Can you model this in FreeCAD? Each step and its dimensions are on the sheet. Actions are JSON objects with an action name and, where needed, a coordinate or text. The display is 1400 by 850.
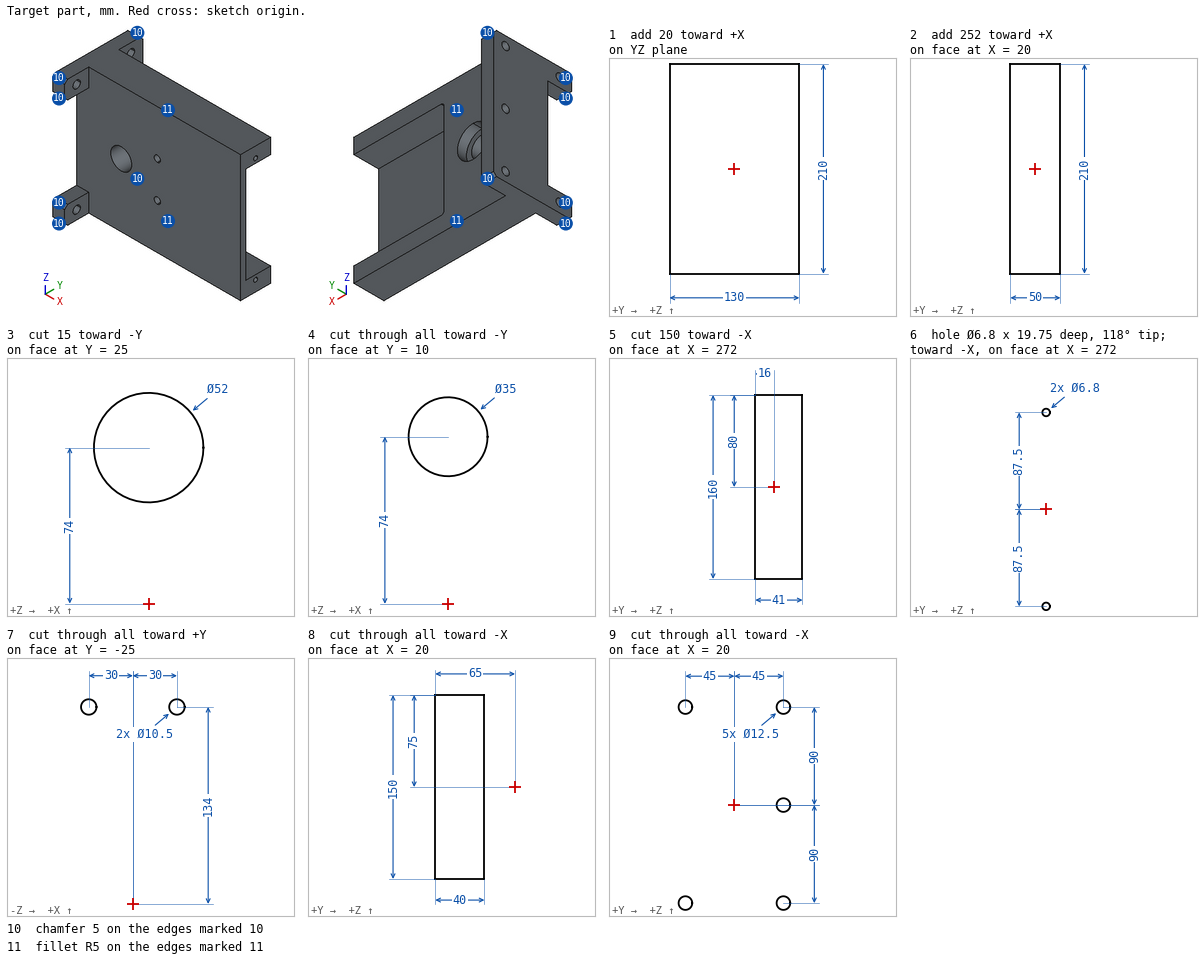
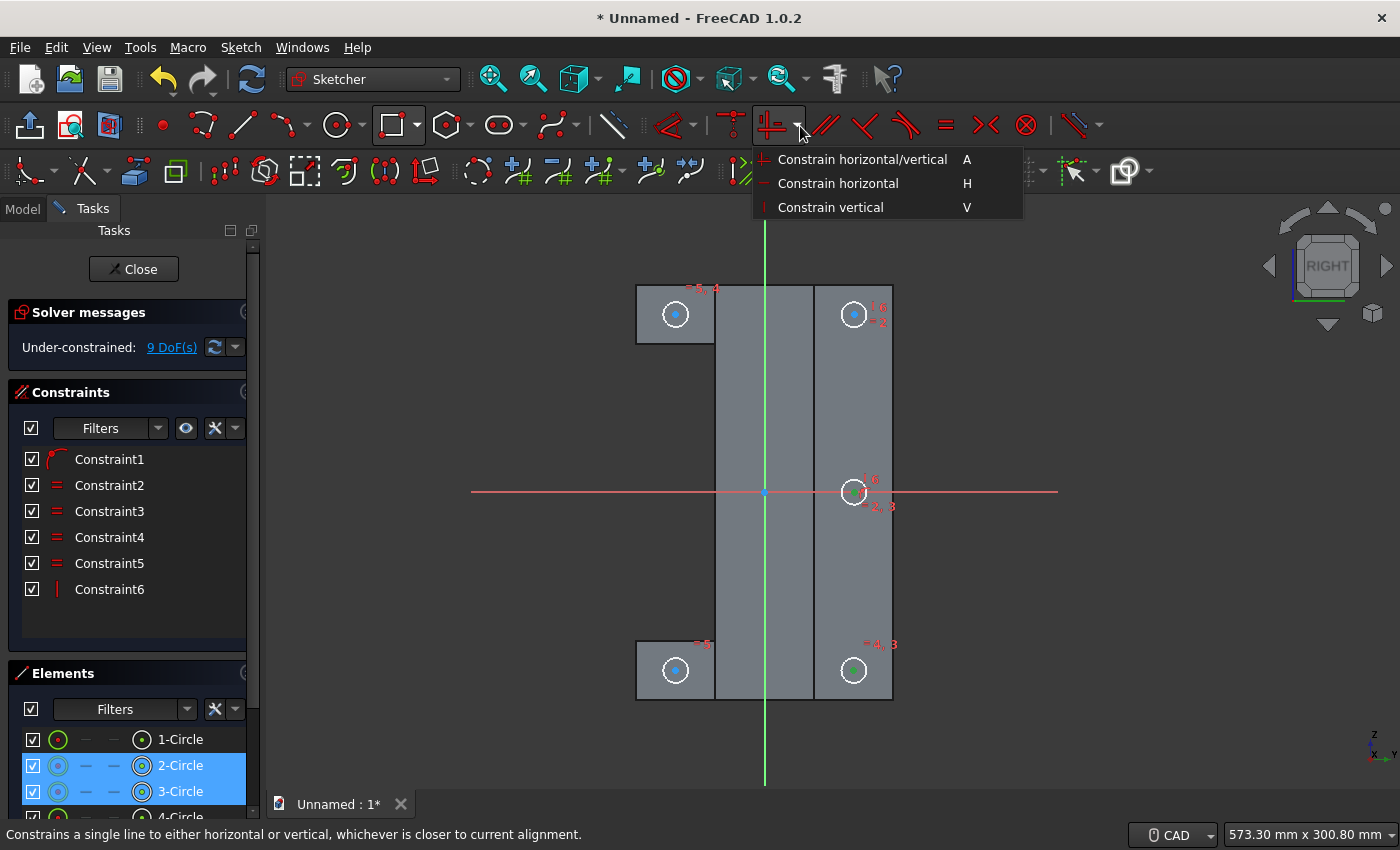
{"action": "left_click", "coordinate": [888, 207]}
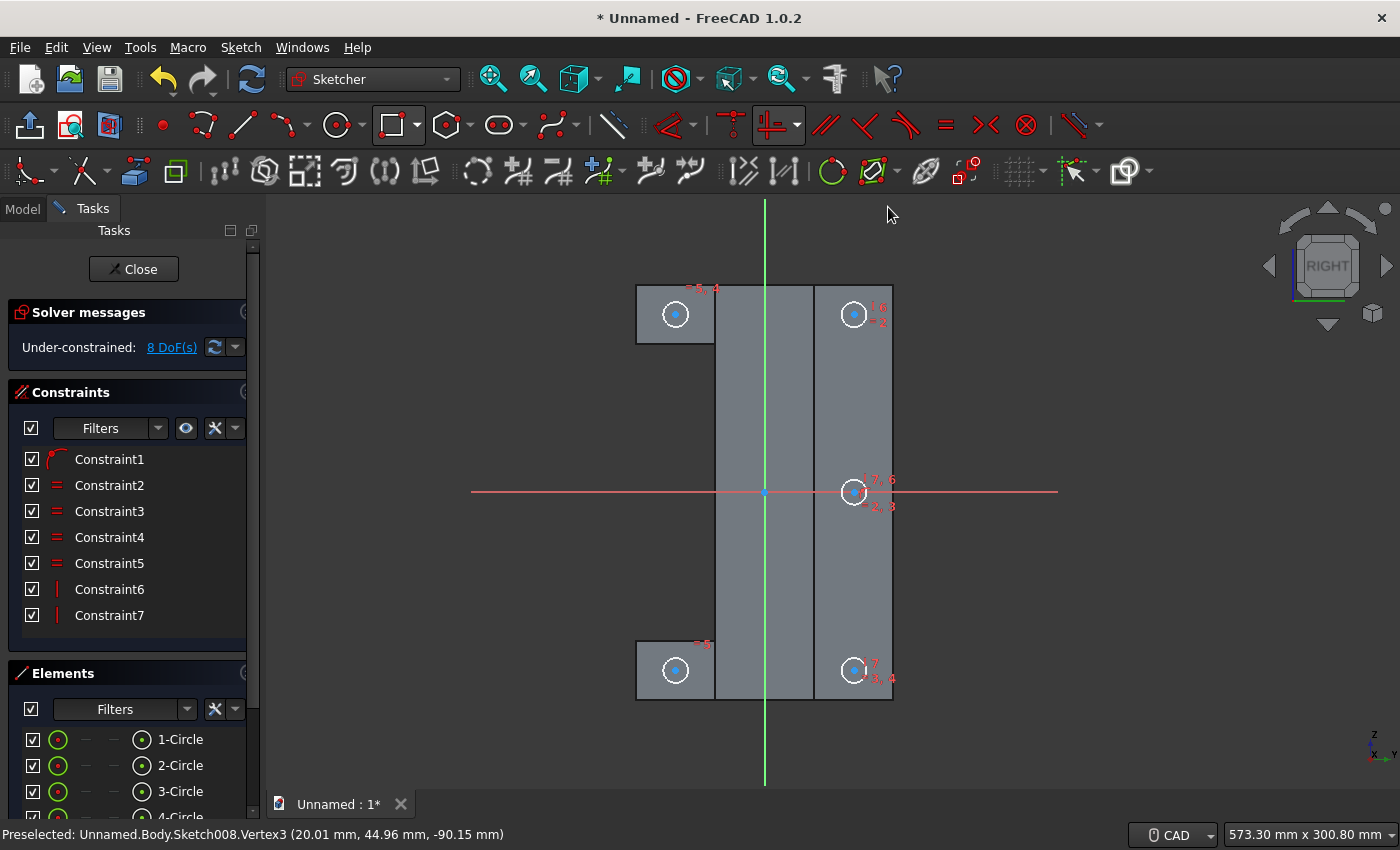
{"action": "left_click", "coordinate": [854, 315]}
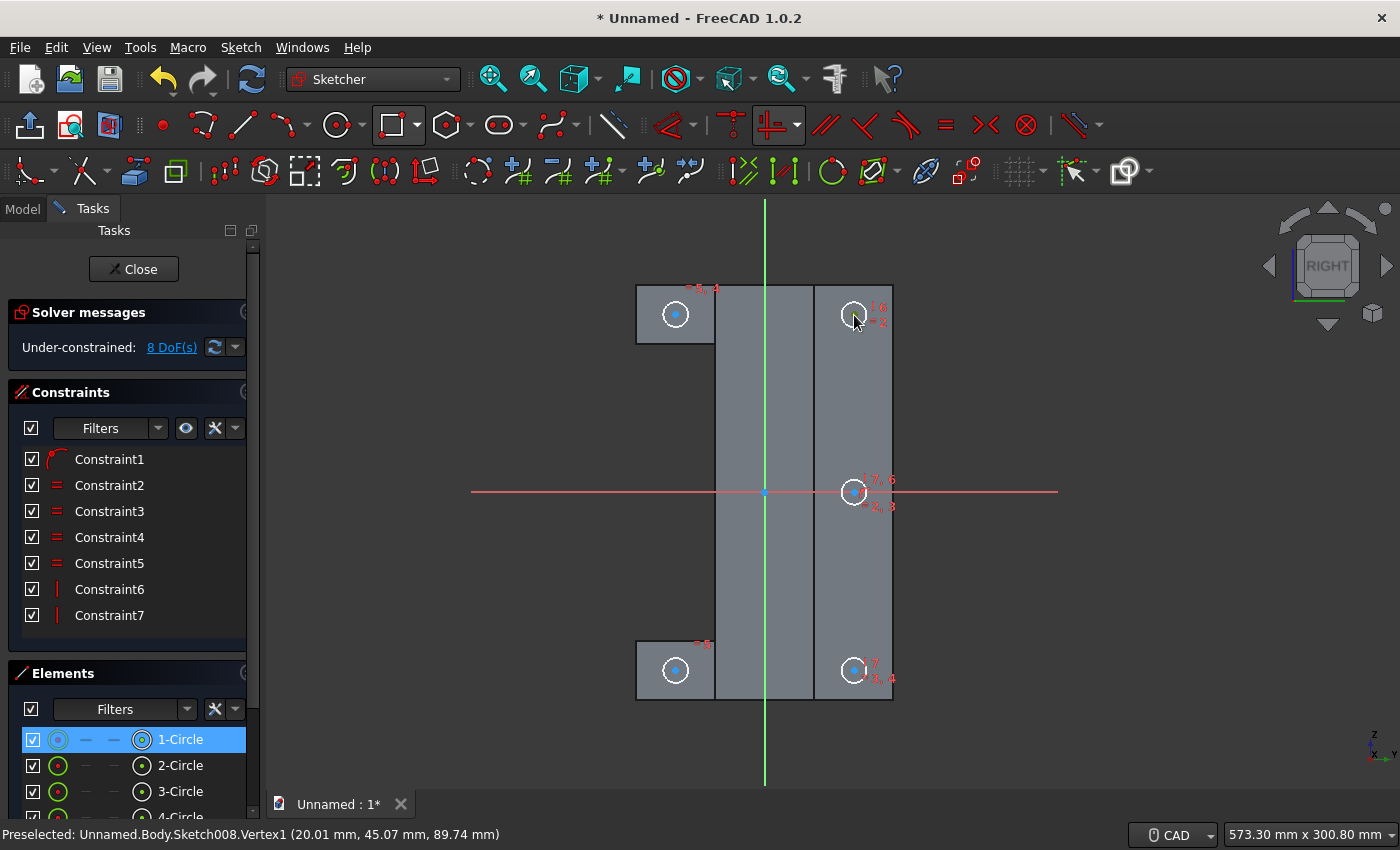
{"action": "left_click", "coordinate": [676, 315]}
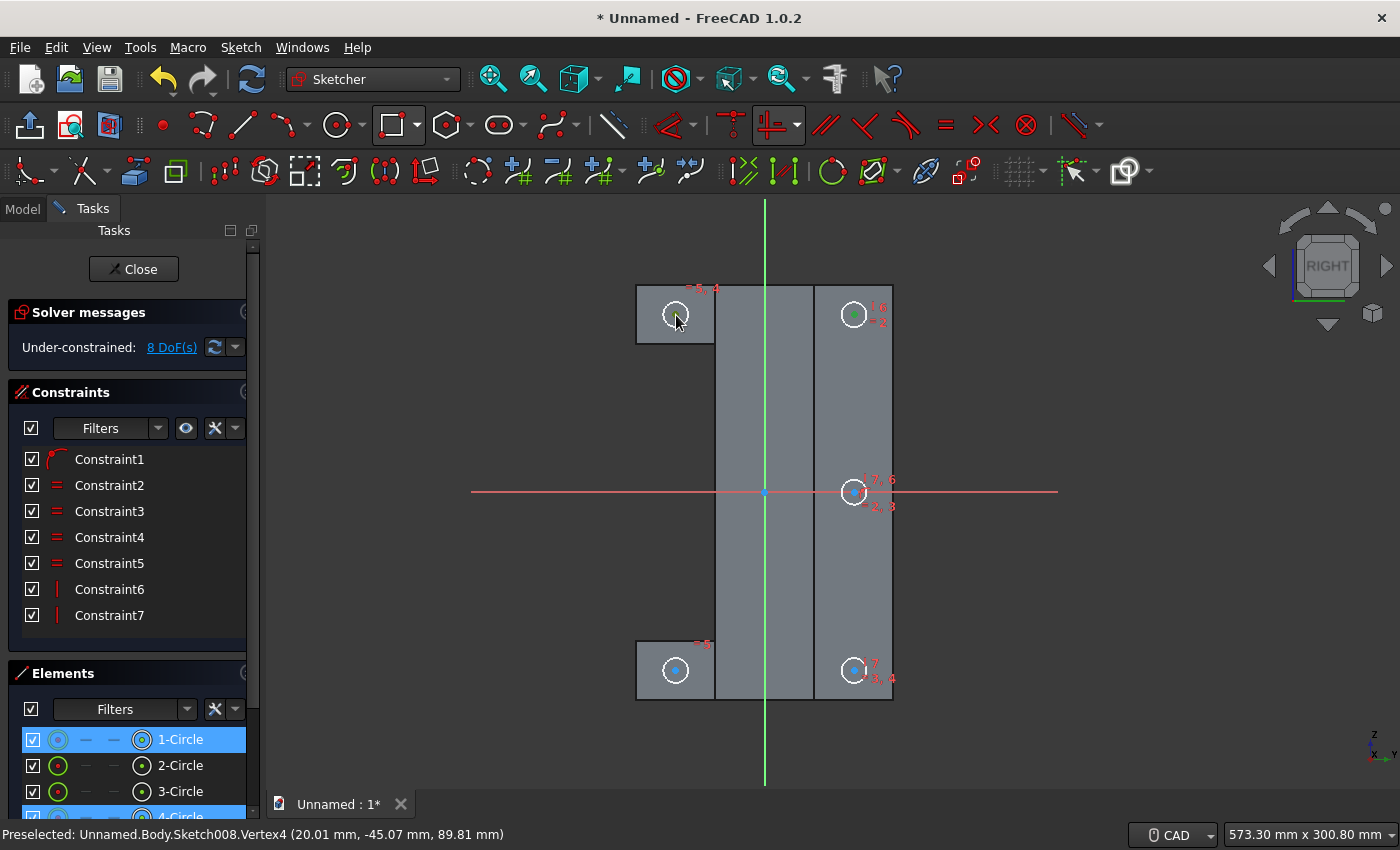
{"action": "left_click", "coordinate": [800, 126]}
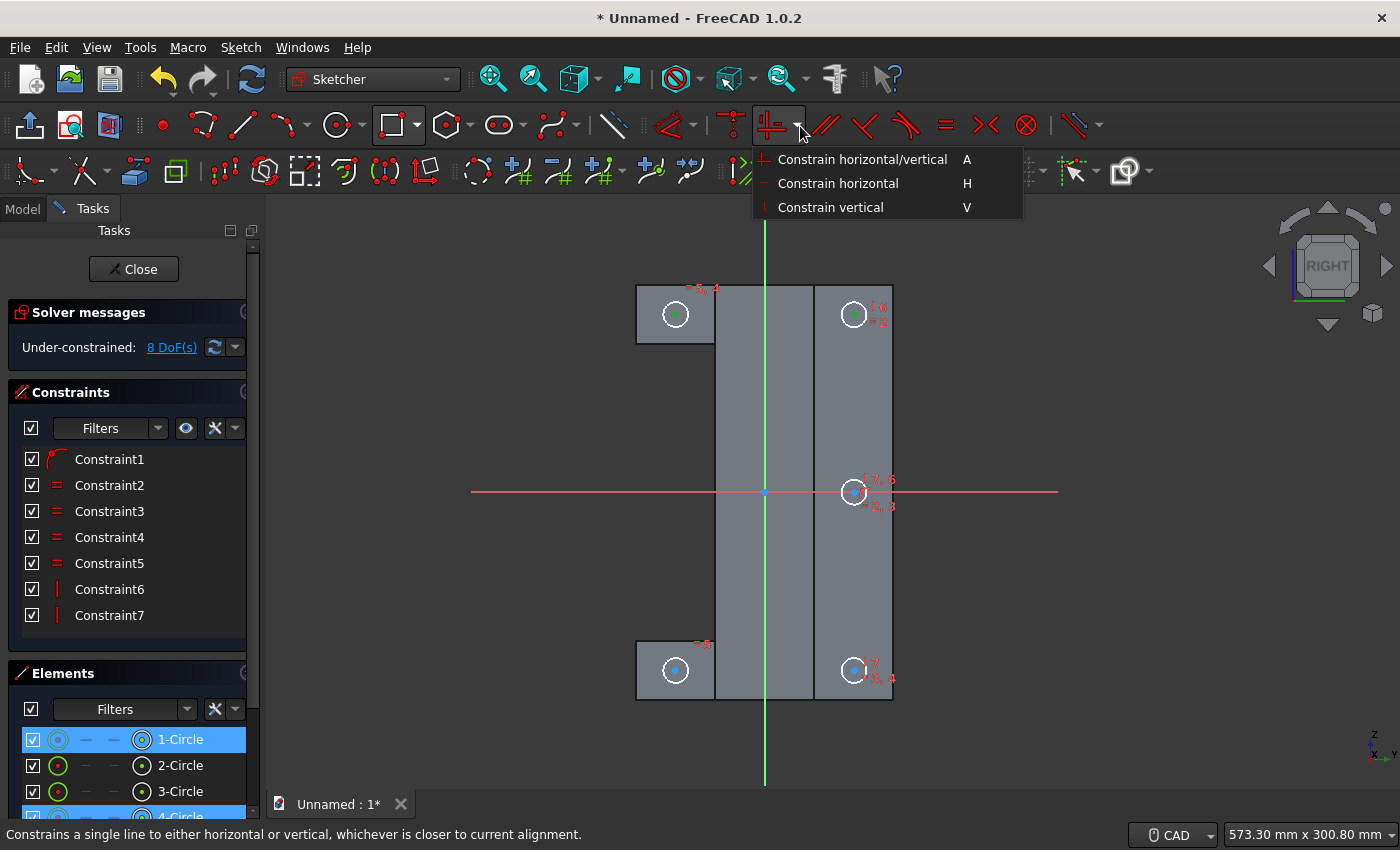
{"action": "left_click", "coordinate": [888, 183]}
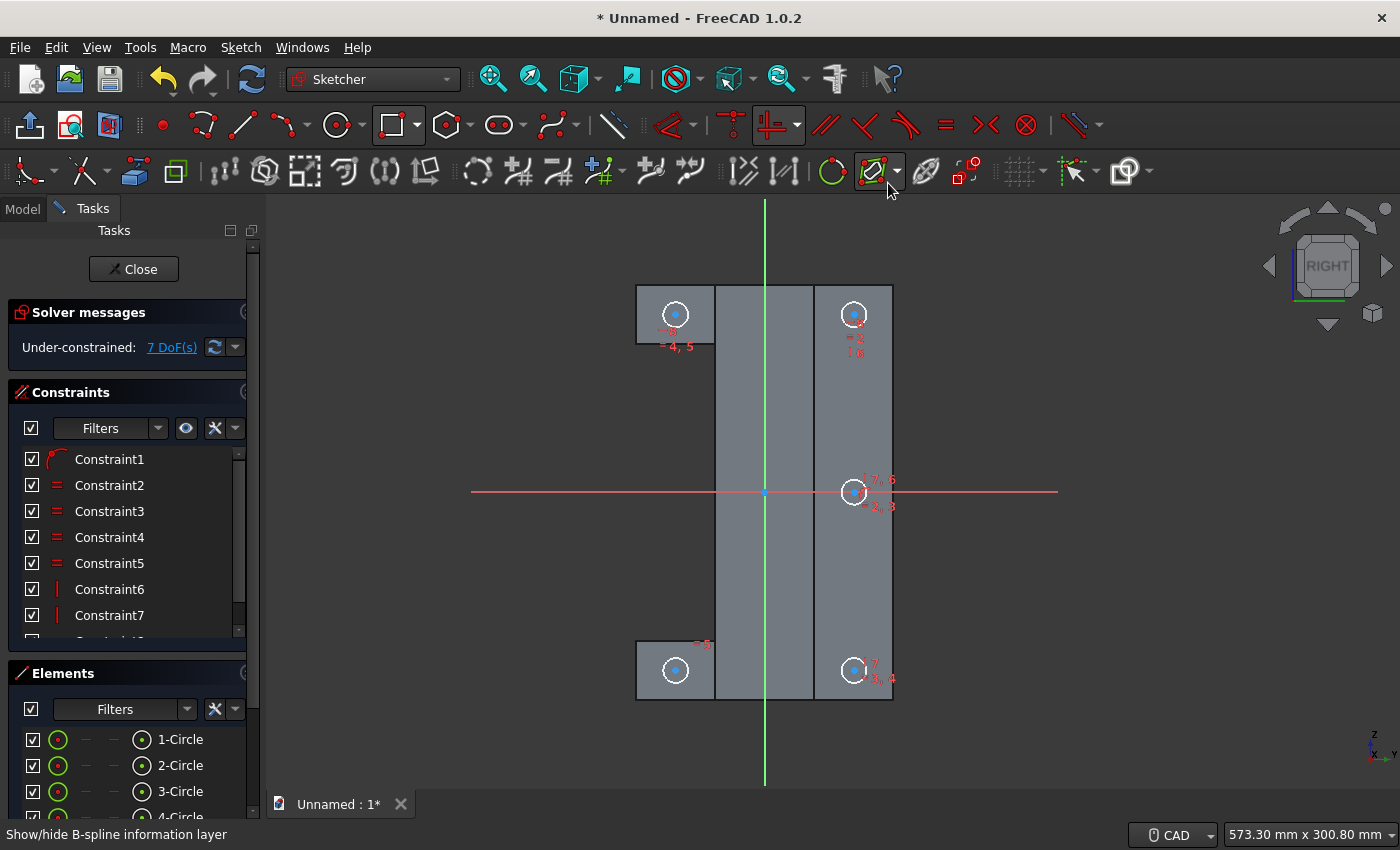
{"action": "left_click", "coordinate": [676, 315]}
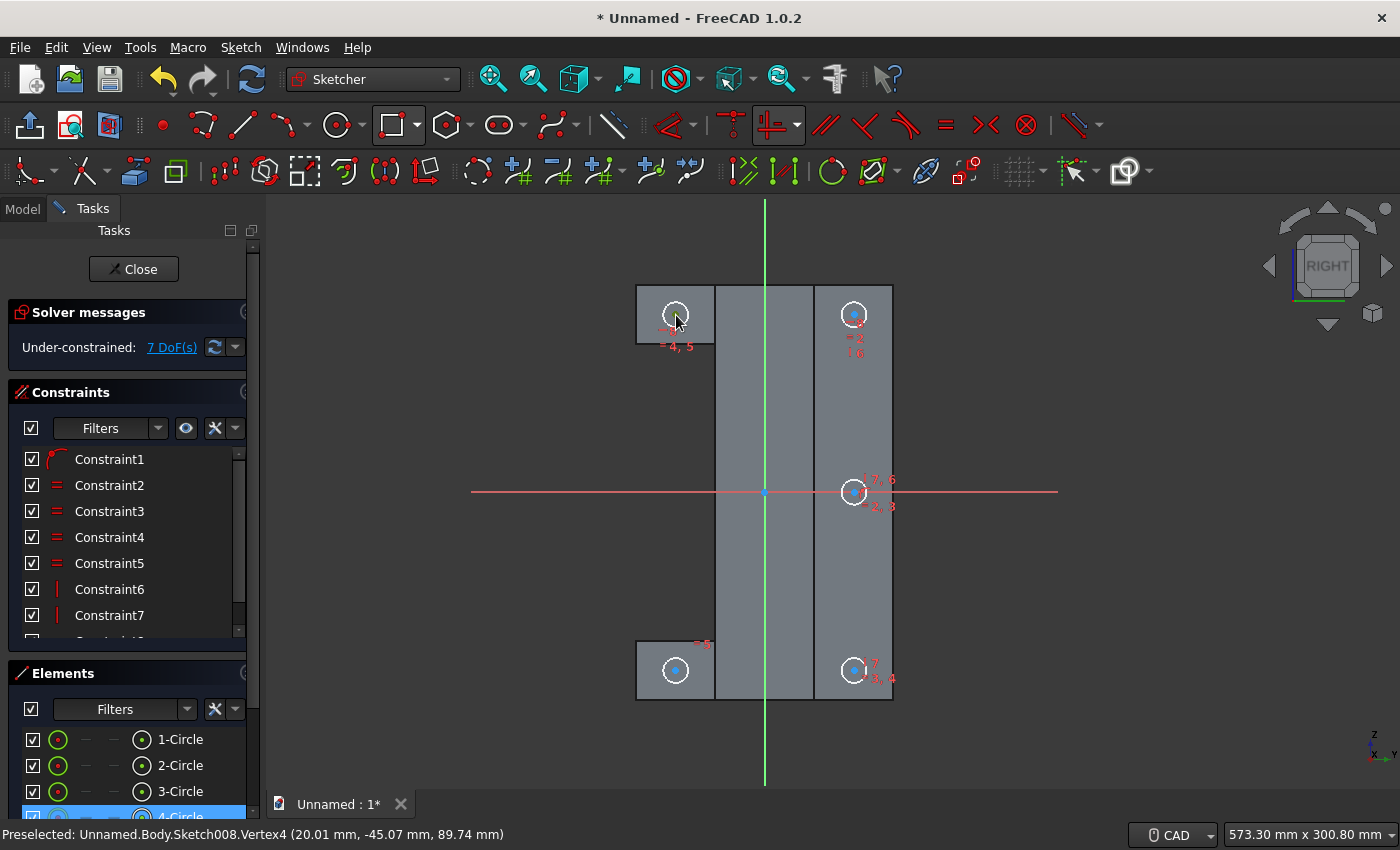
{"action": "left_click", "coordinate": [676, 671]}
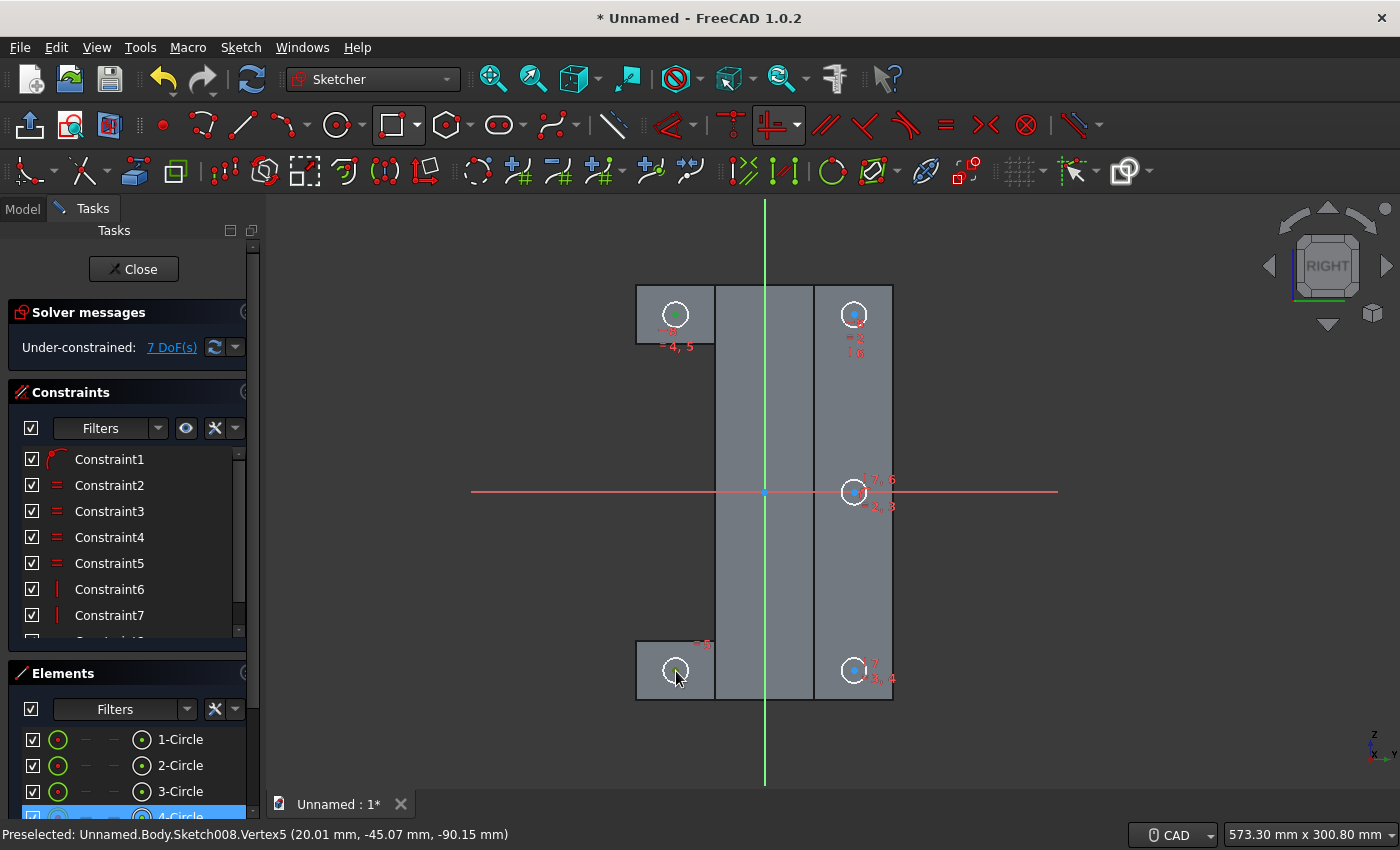
{"action": "left_click", "coordinate": [800, 126]}